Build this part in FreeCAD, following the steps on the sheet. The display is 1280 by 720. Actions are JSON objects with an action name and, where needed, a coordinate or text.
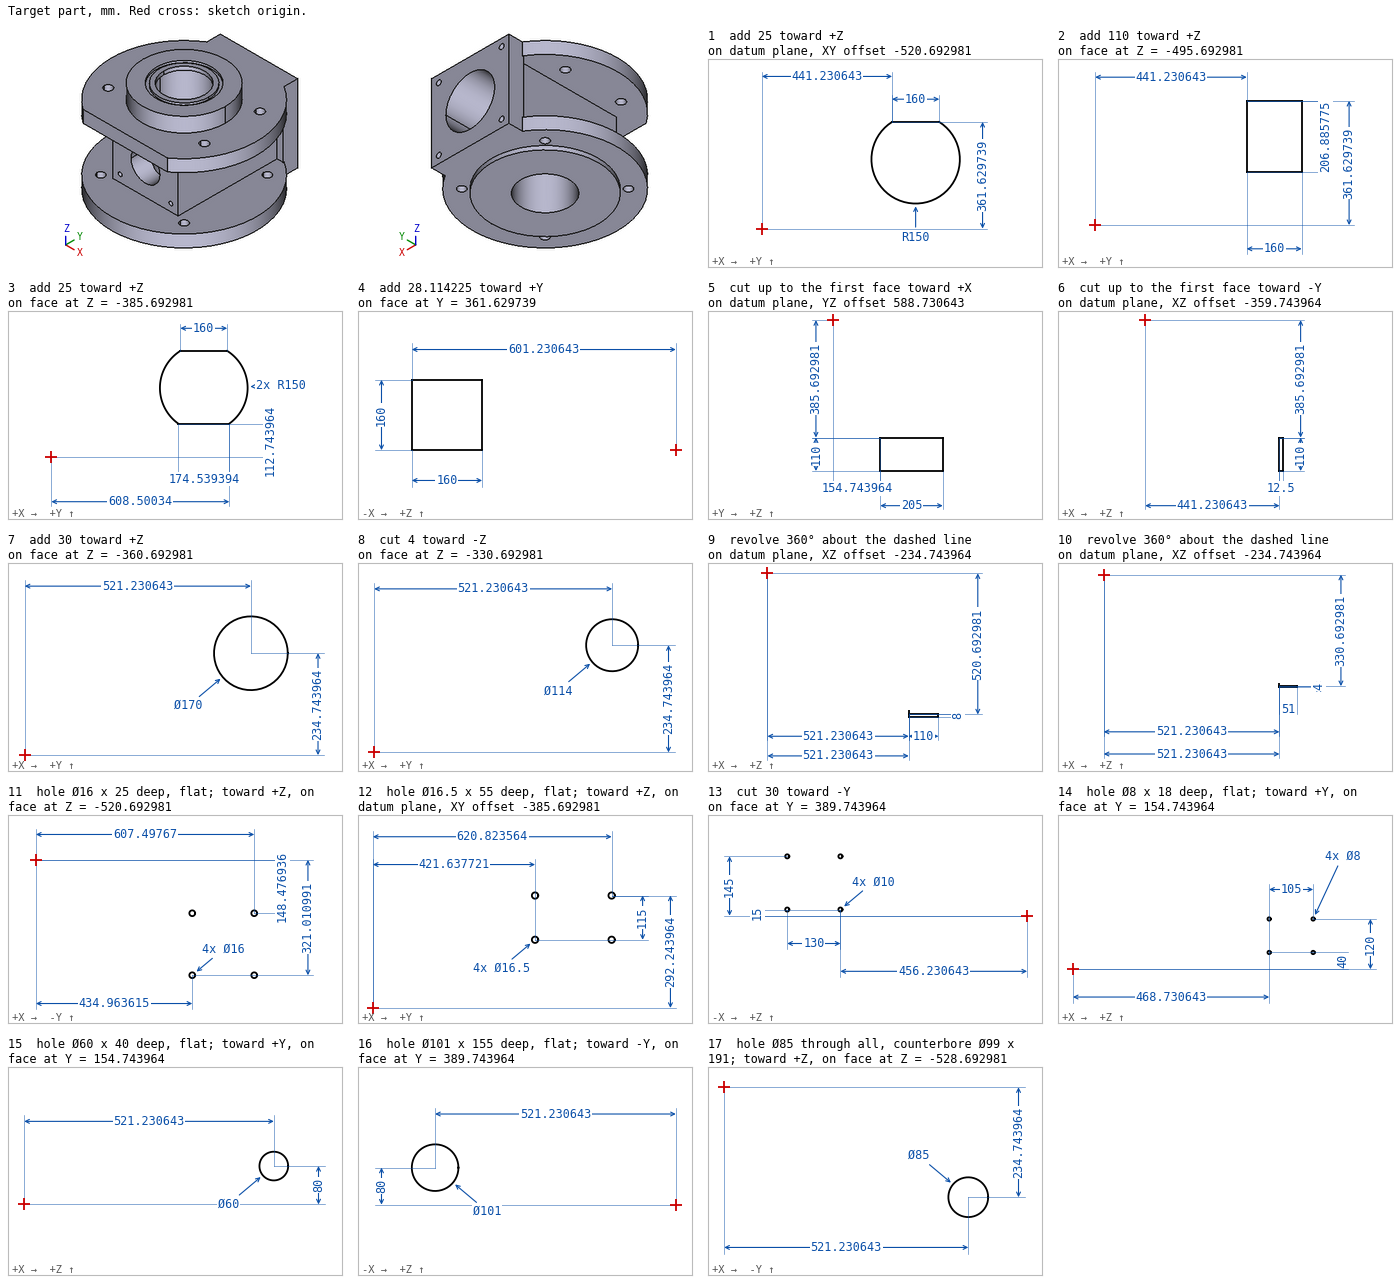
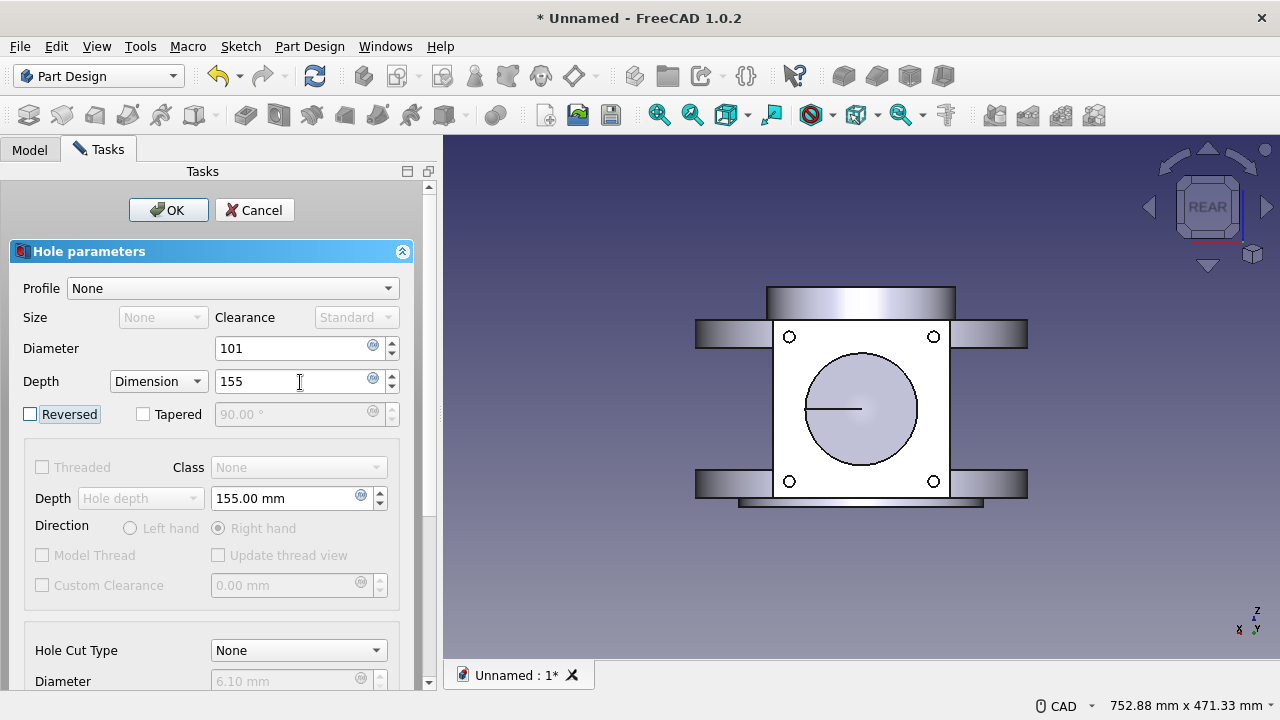
{"action": "scroll", "coordinate": [429, 436], "scroll_direction": "down", "scroll_amount": 4}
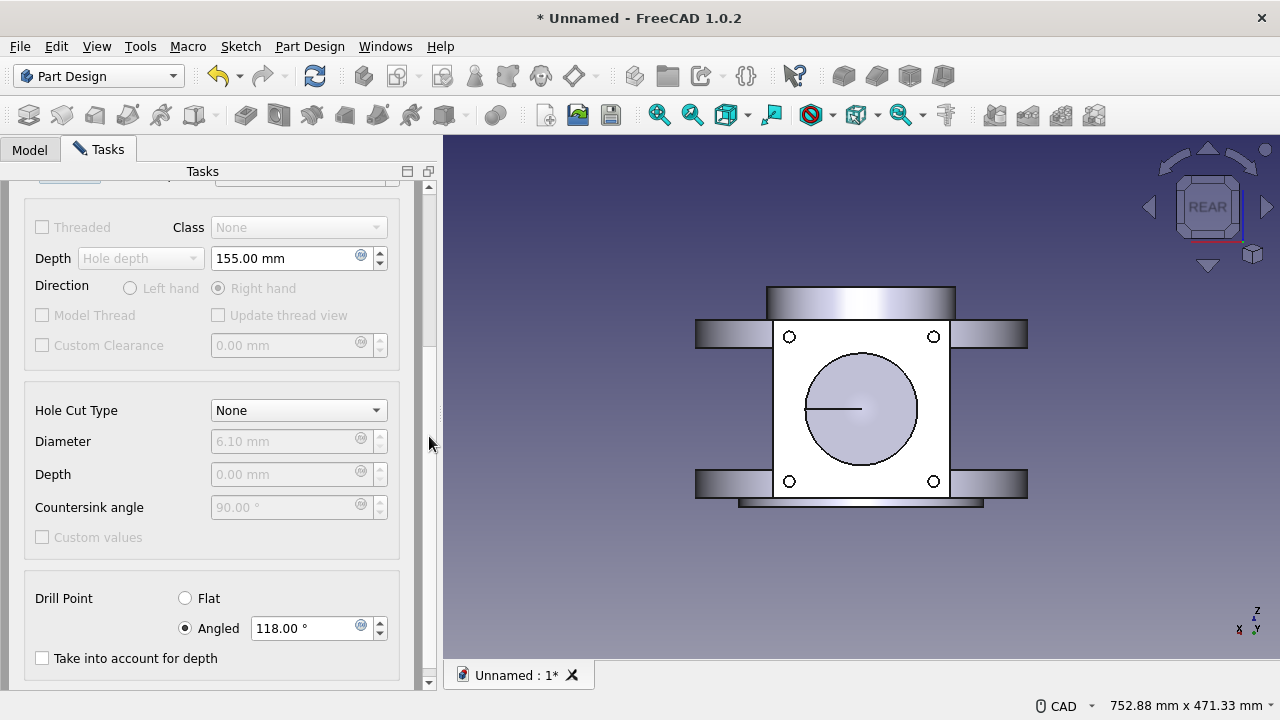
{"action": "left_click", "coordinate": [186, 596]}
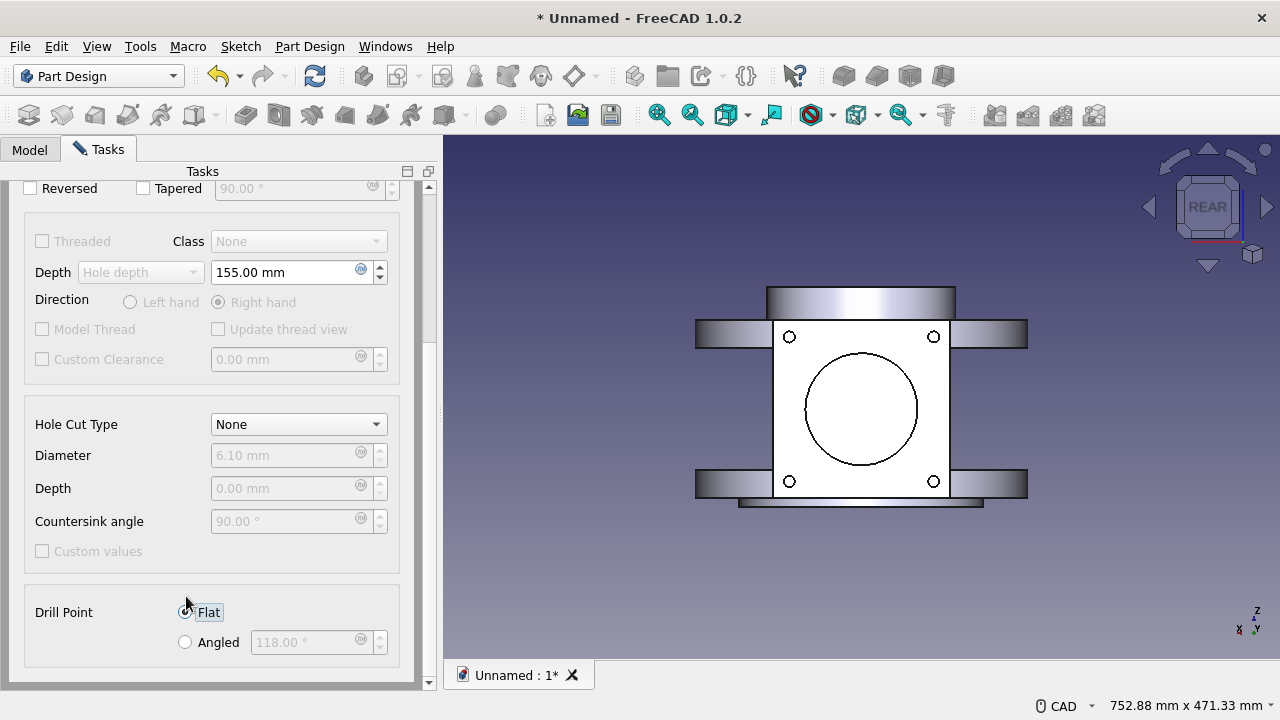
{"action": "scroll", "coordinate": [429, 436], "scroll_direction": "up", "scroll_amount": 5}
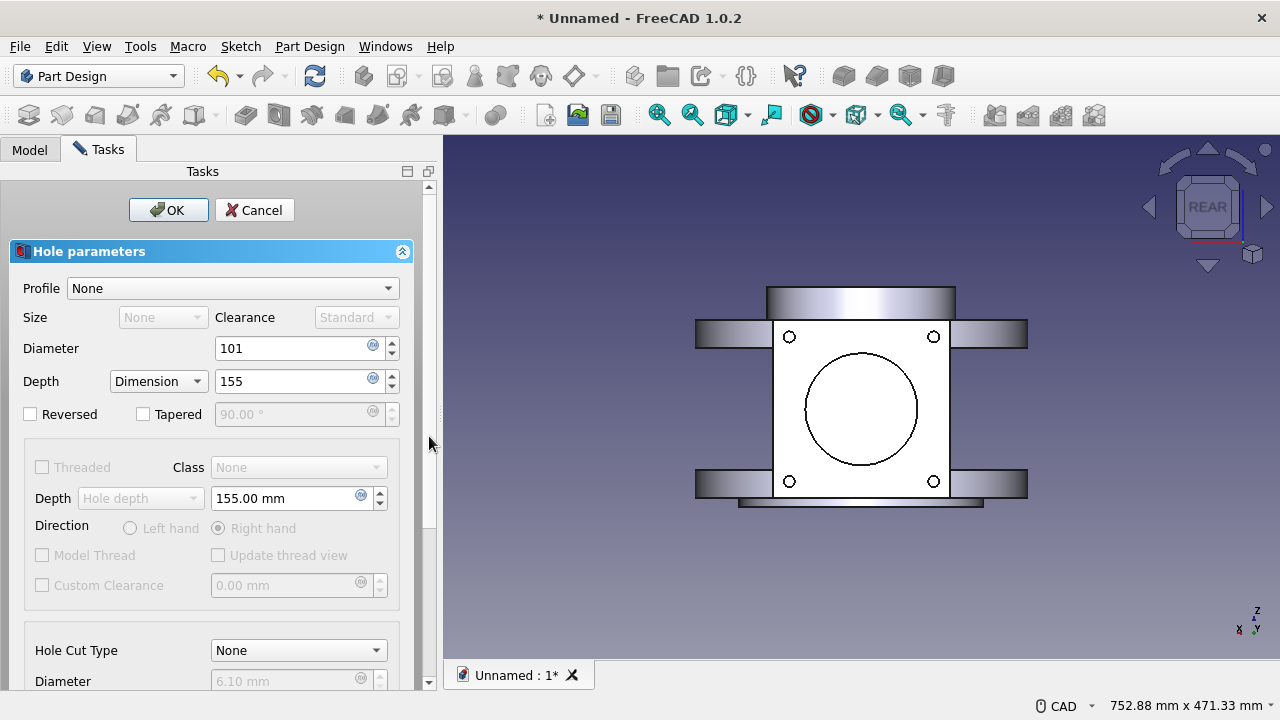
{"action": "left_click", "coordinate": [169, 210]}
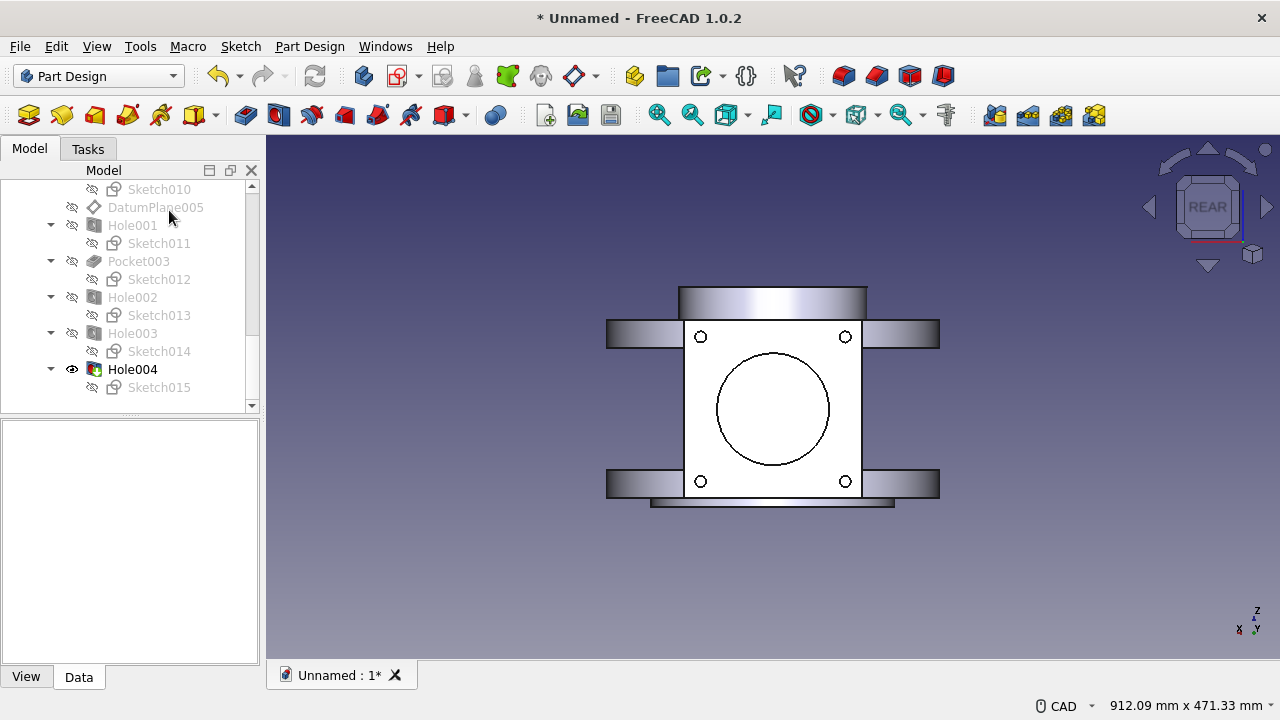
{"action": "left_click", "coordinate": [660, 116]}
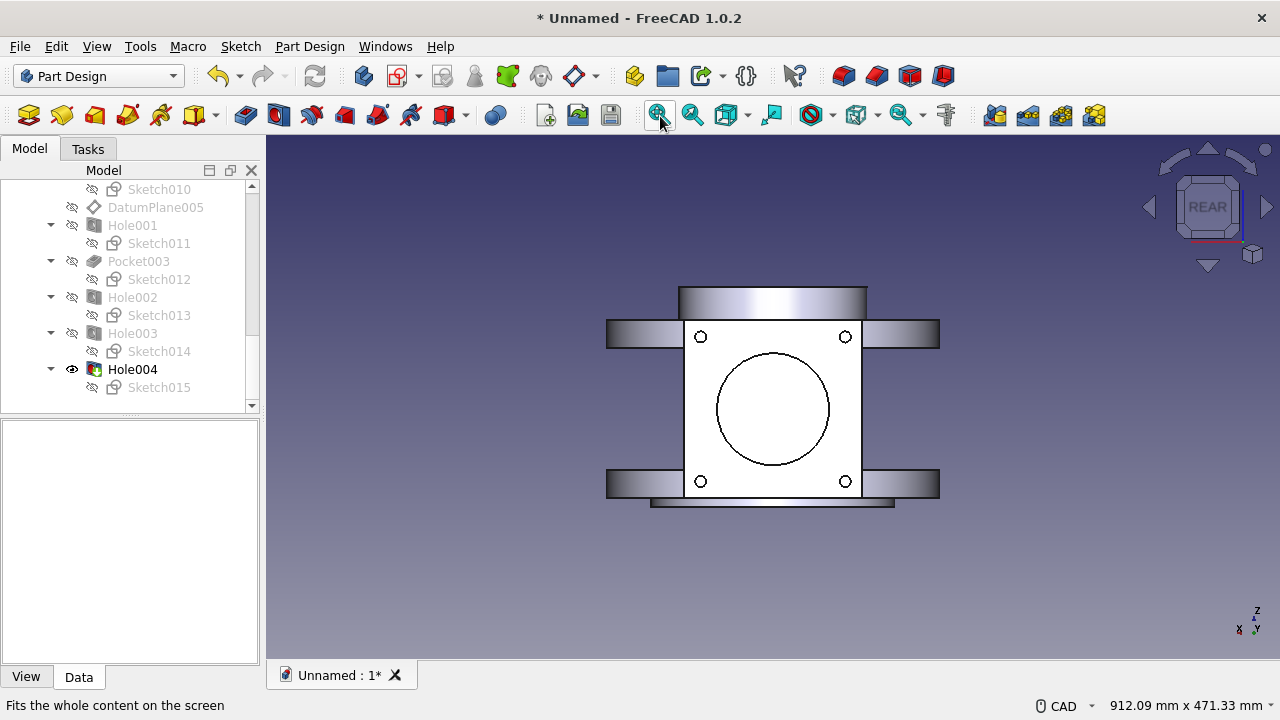
{"action": "key", "text": "5"}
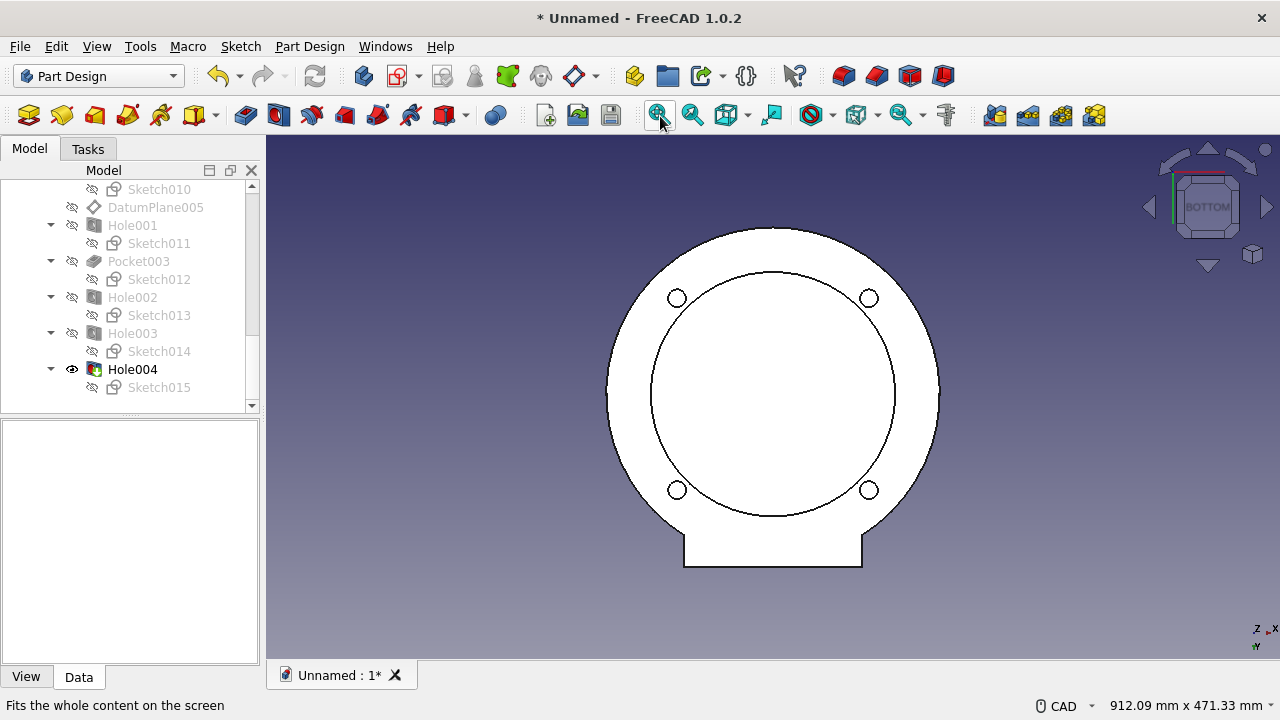
{"action": "left_click", "coordinate": [773, 393]}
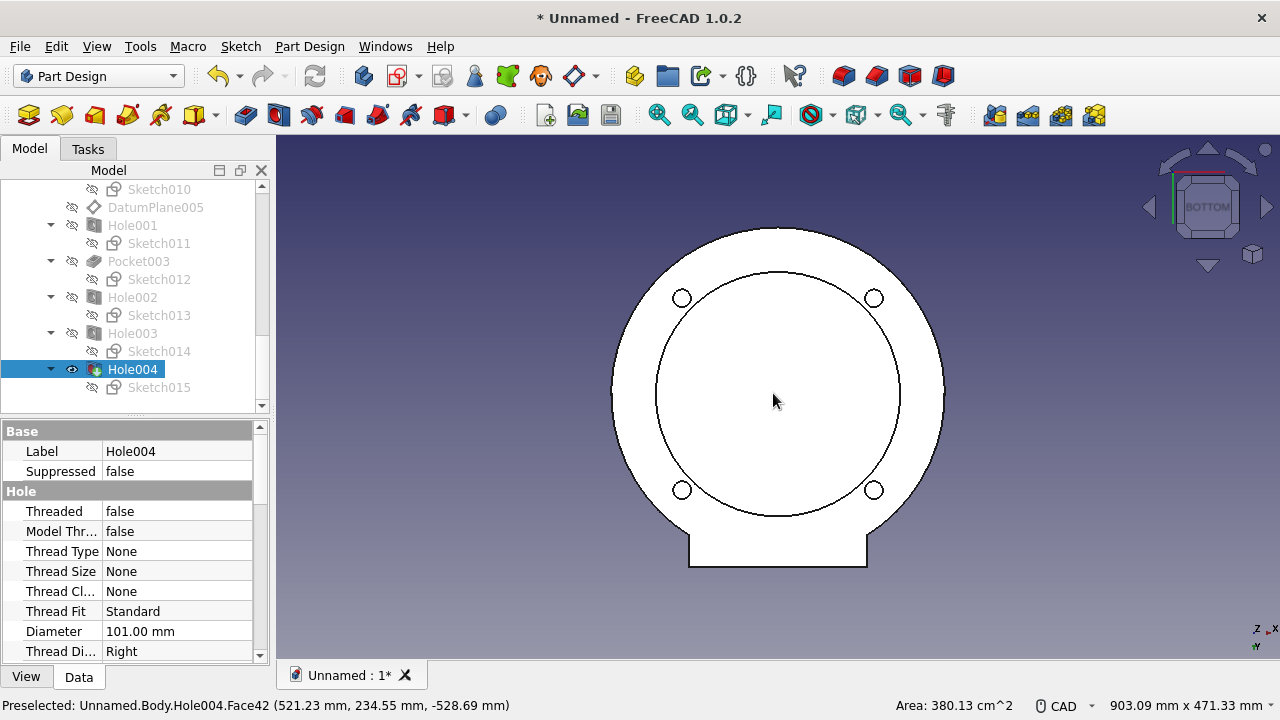
{"action": "left_click", "coordinate": [396, 76]}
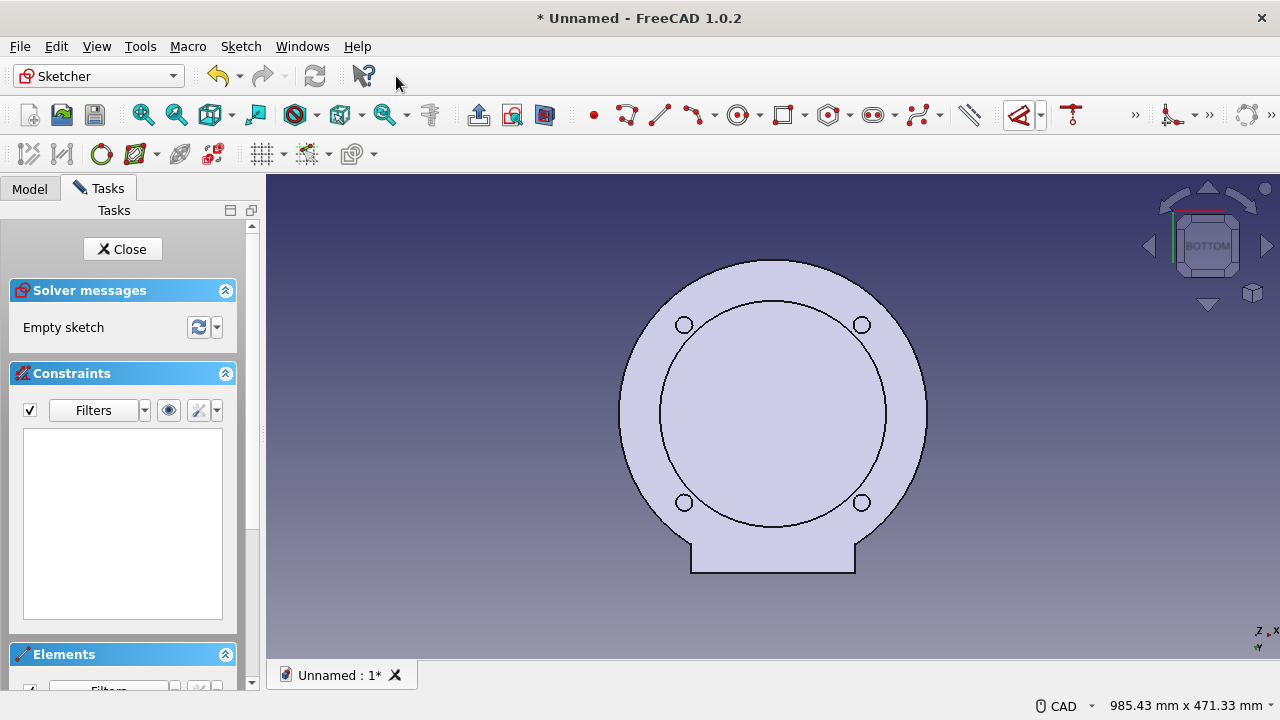
{"action": "scroll", "coordinate": [803, 413], "scroll_direction": "up", "scroll_amount": 6}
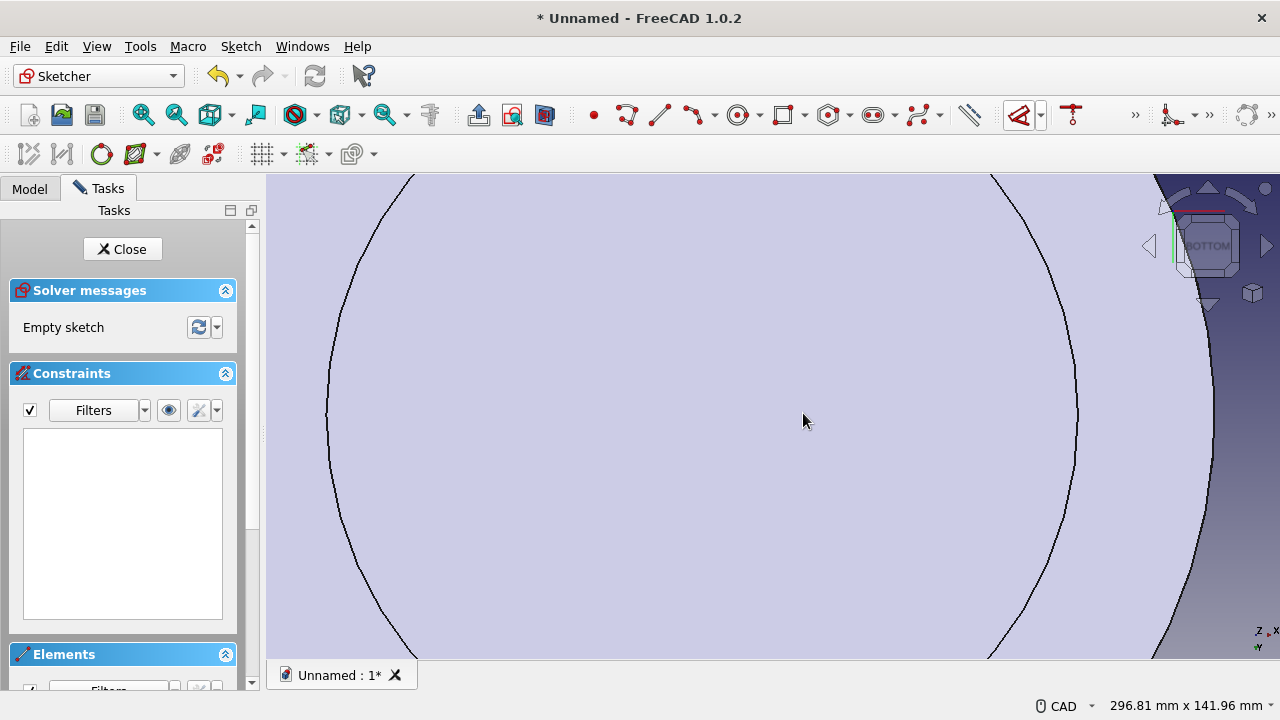
{"action": "left_click", "coordinate": [738, 116]}